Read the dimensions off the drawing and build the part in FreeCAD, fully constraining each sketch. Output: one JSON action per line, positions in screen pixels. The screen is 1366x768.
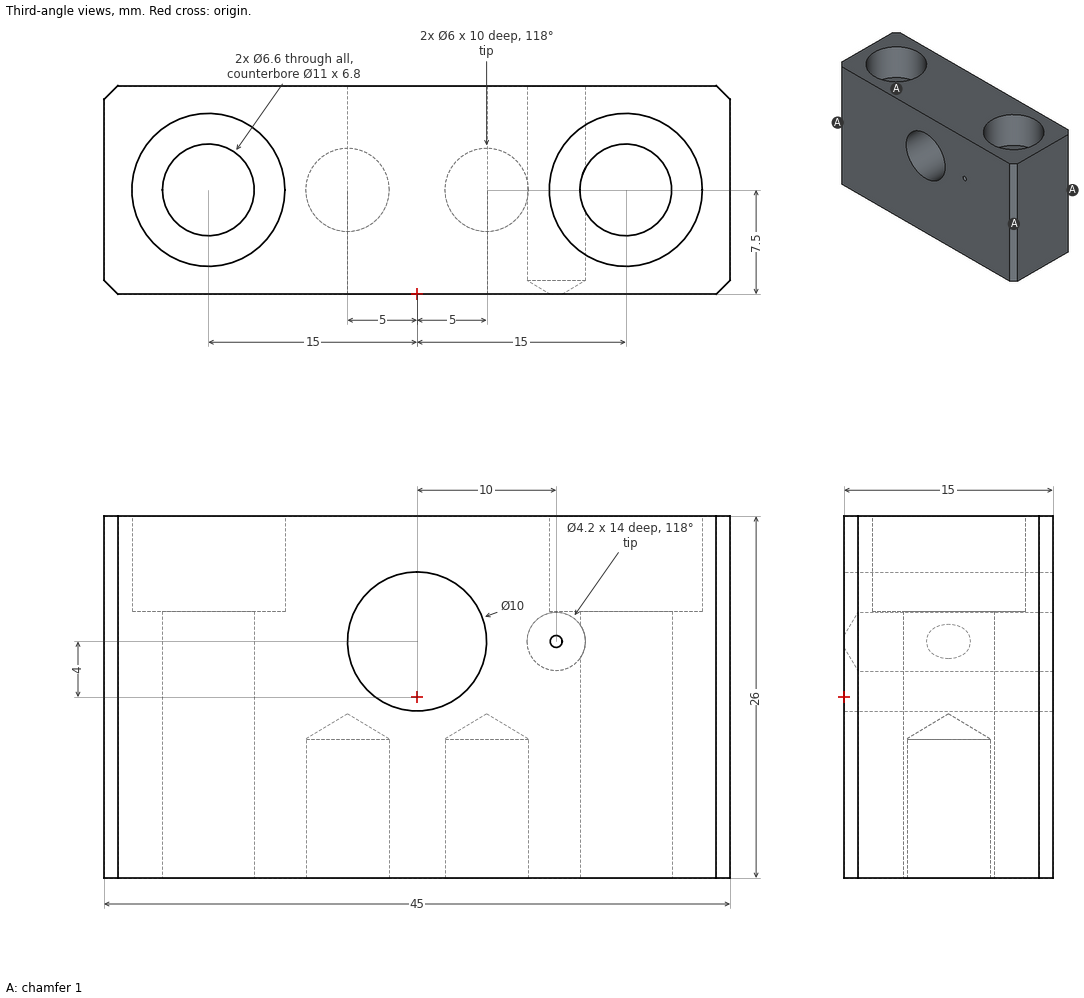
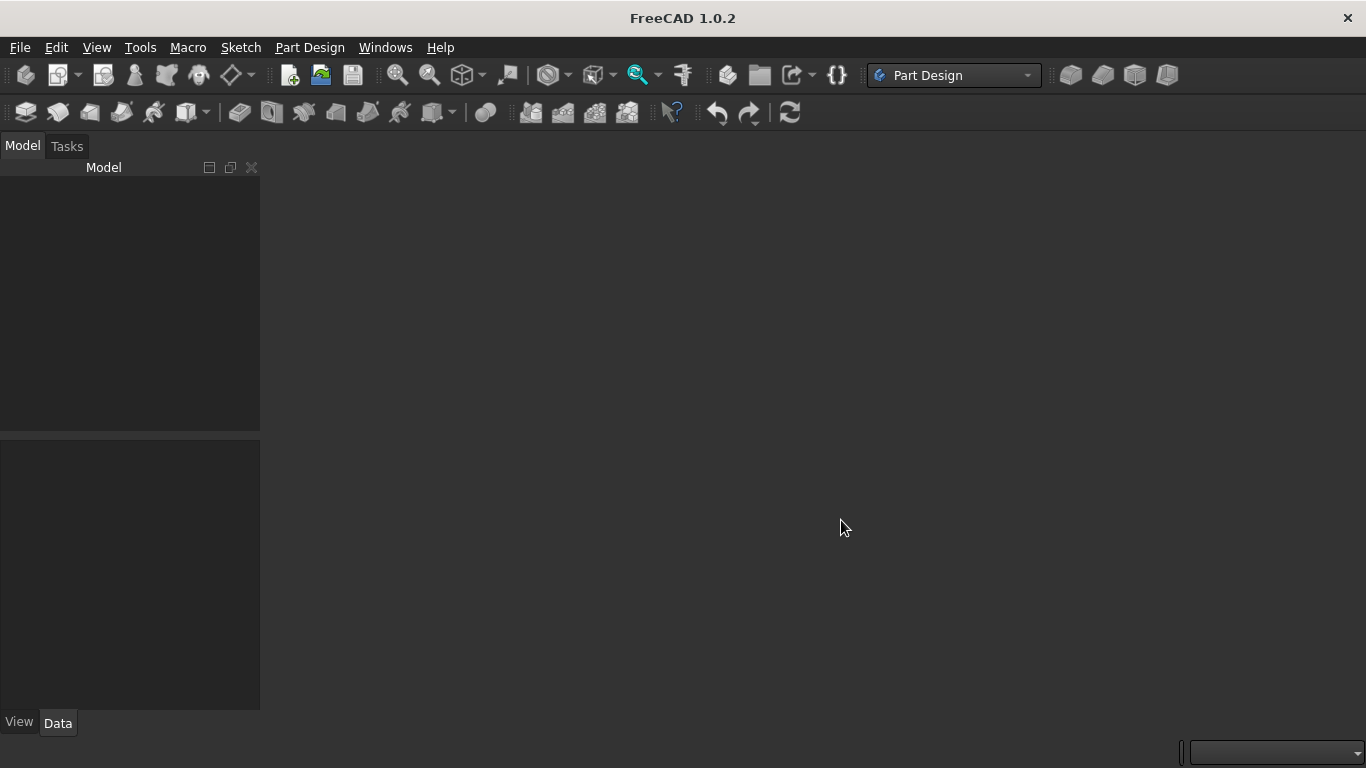
{"action": "left_click", "coordinate": [290, 76]}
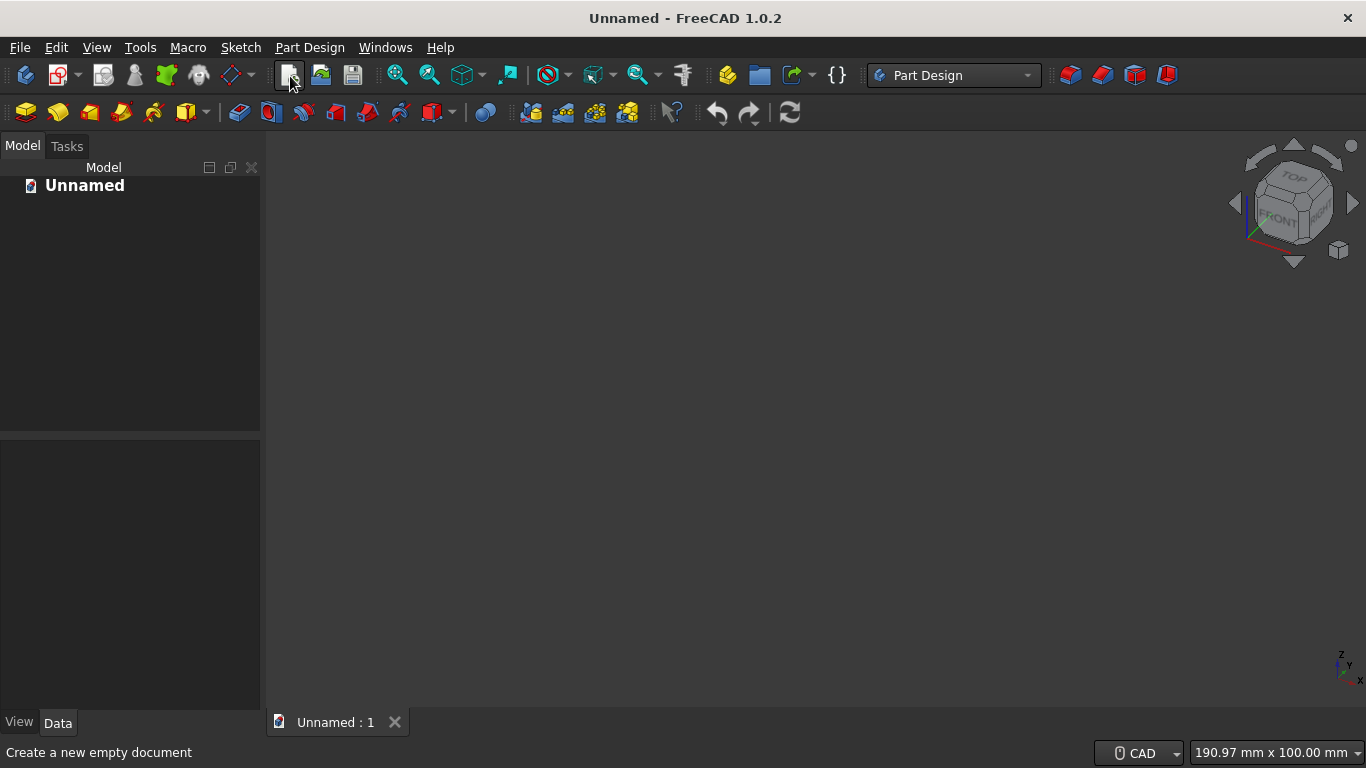
{"action": "left_click", "coordinate": [58, 76]}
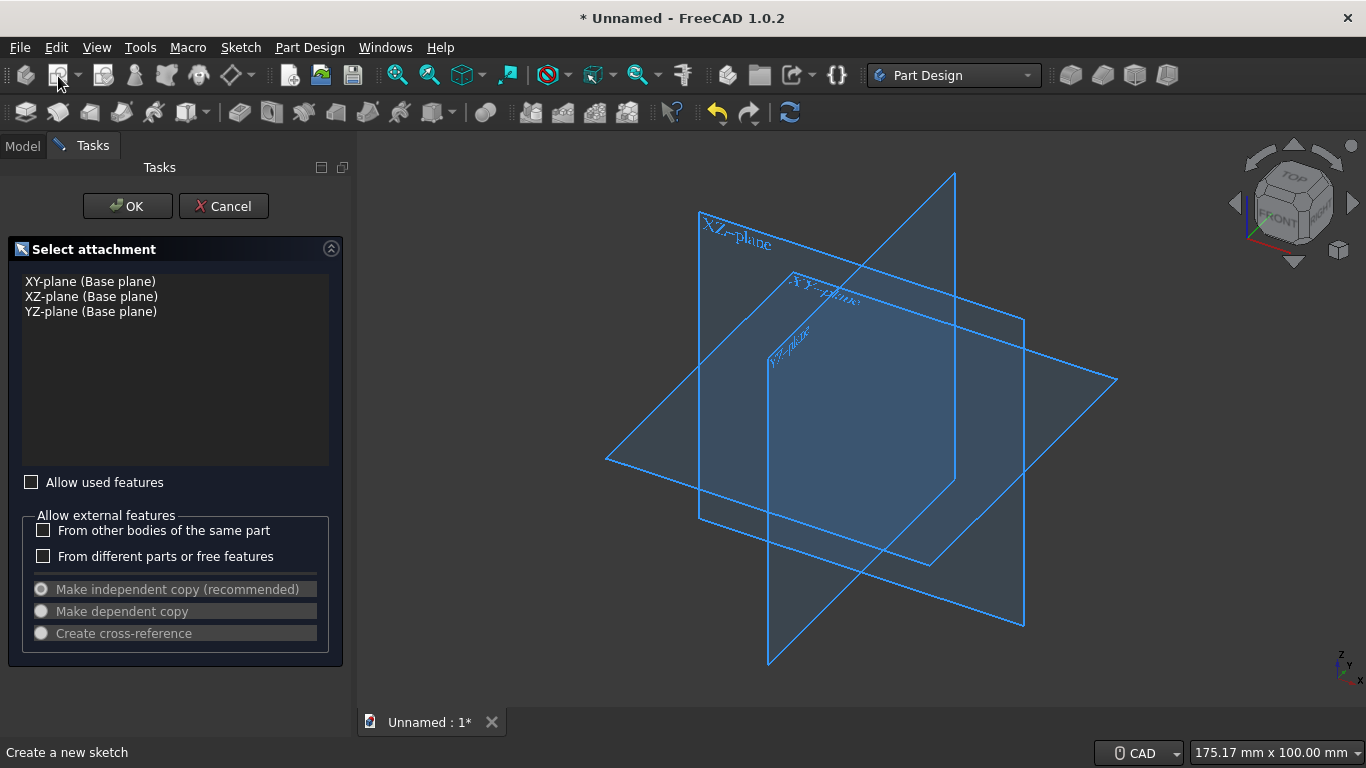
{"action": "left_click", "coordinate": [82, 296]}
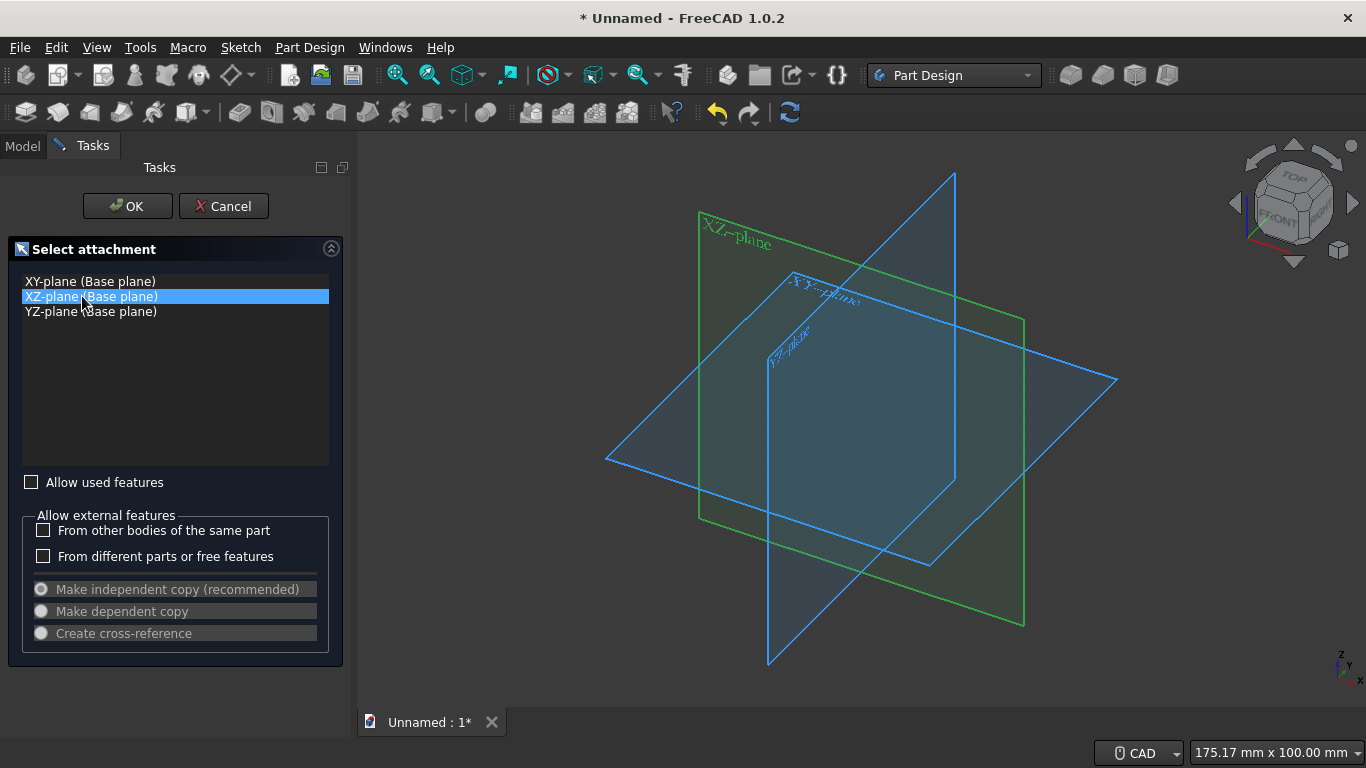
{"action": "left_click", "coordinate": [128, 206]}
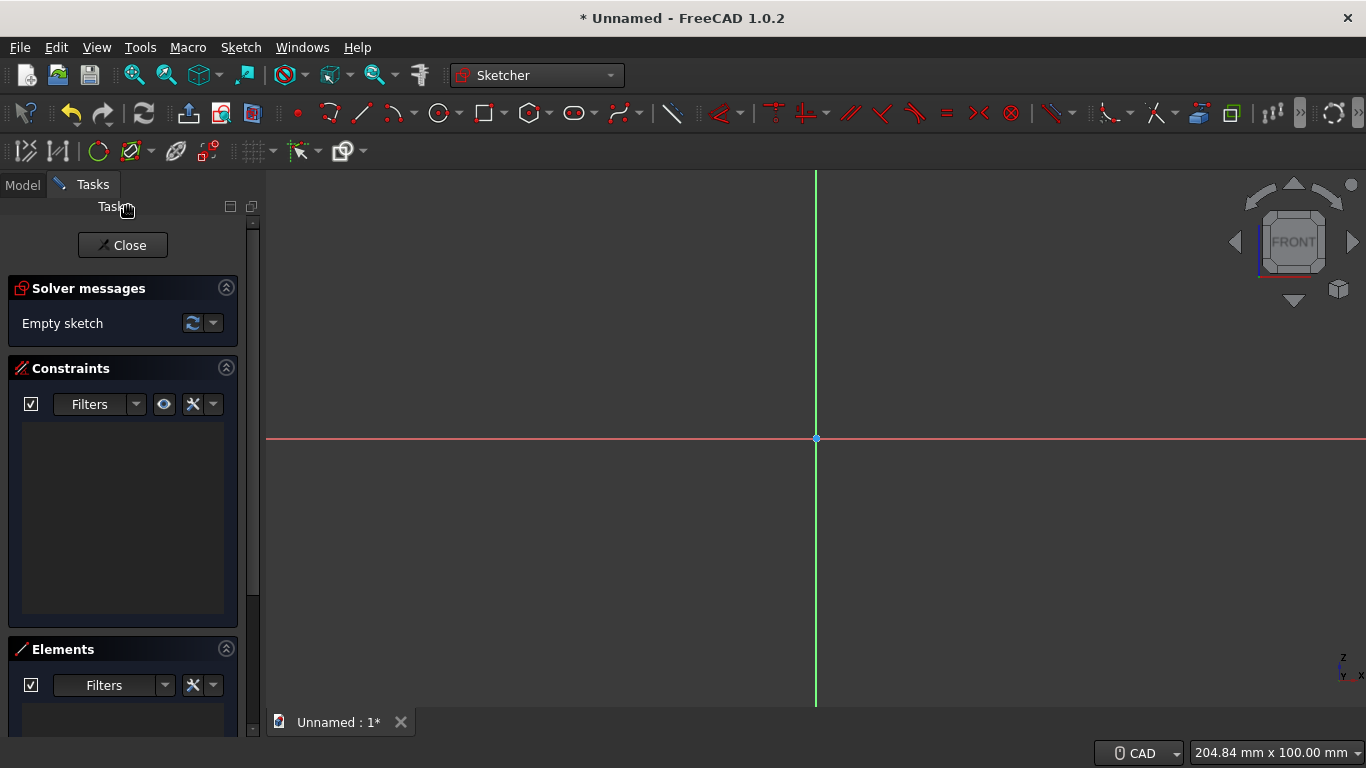
{"action": "scroll", "coordinate": [872, 438], "scroll_direction": "up", "scroll_amount": 4}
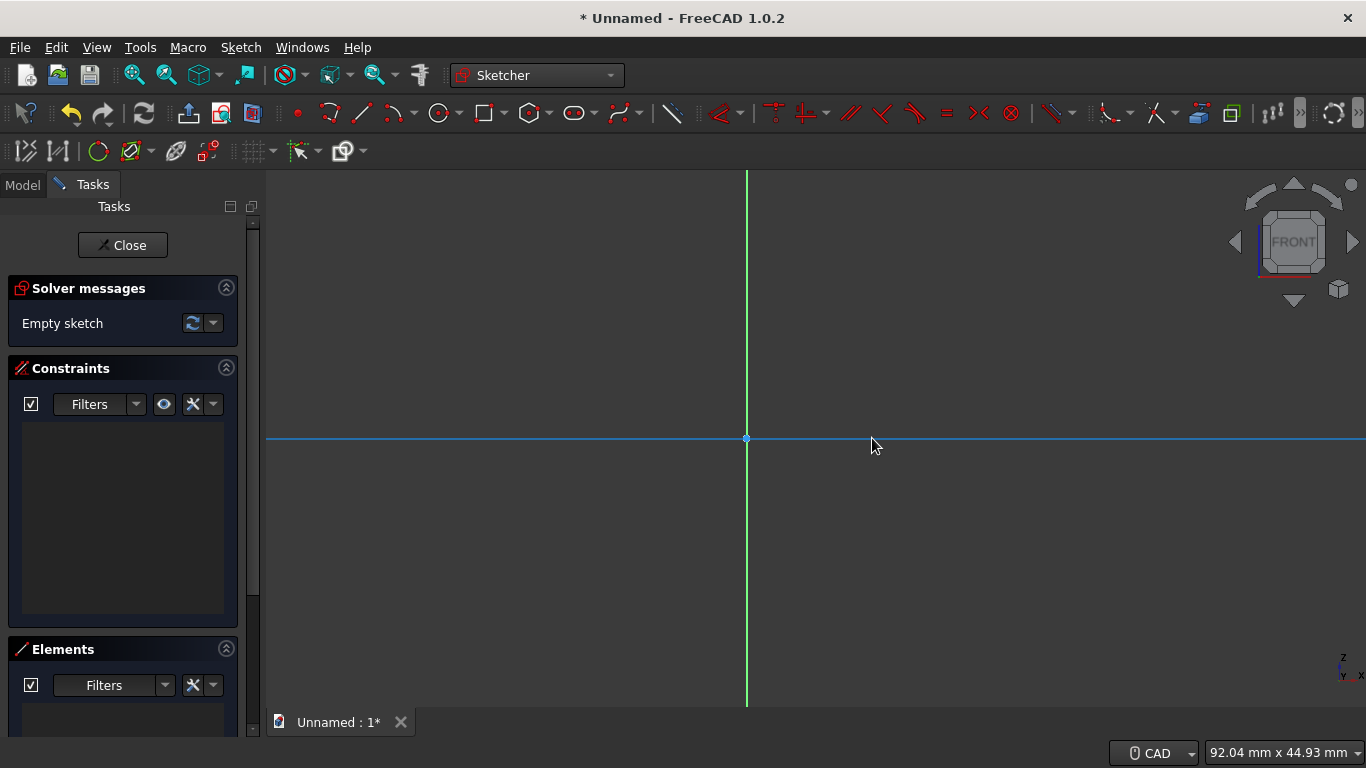
{"action": "key", "text": "g v"}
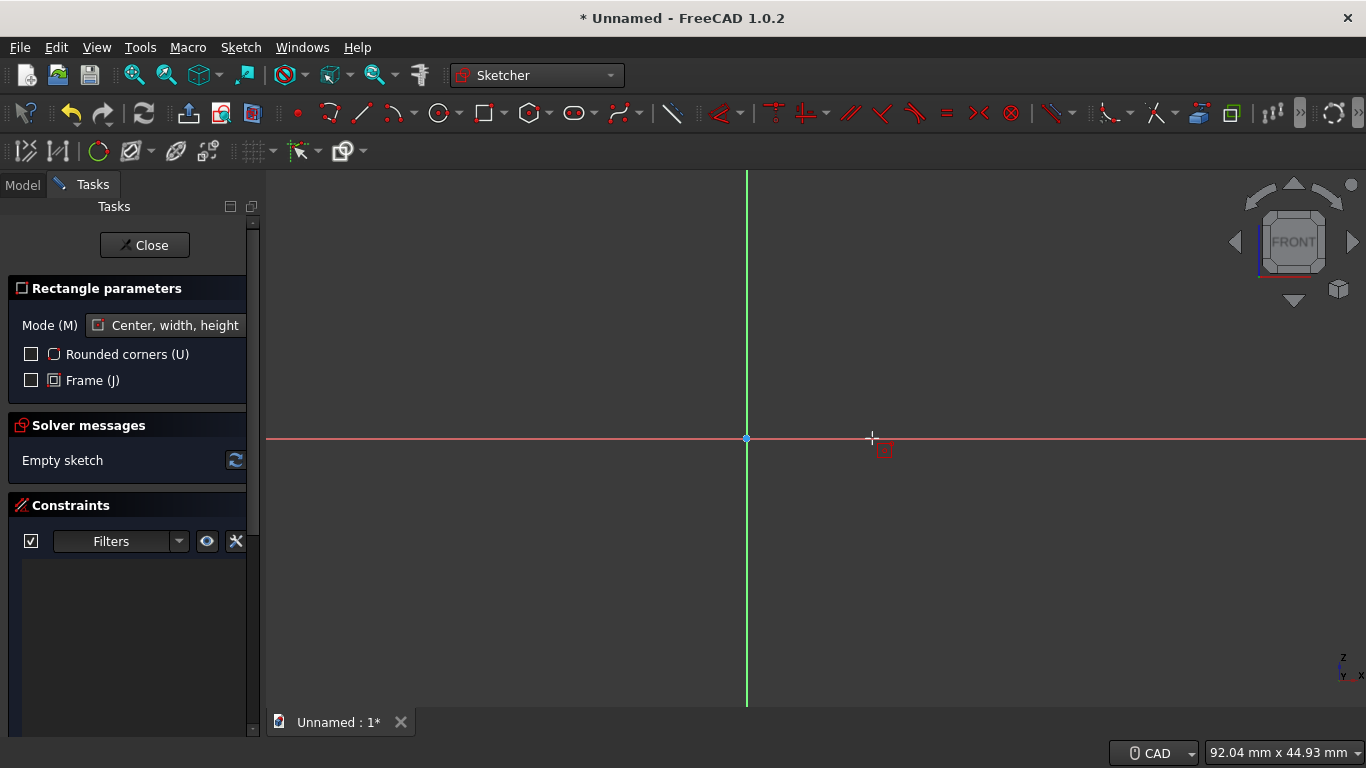
{"action": "left_click", "coordinate": [747, 438]}
{"action": "left_click", "coordinate": [1016, 283]}
{"action": "key", "text": "Escape"}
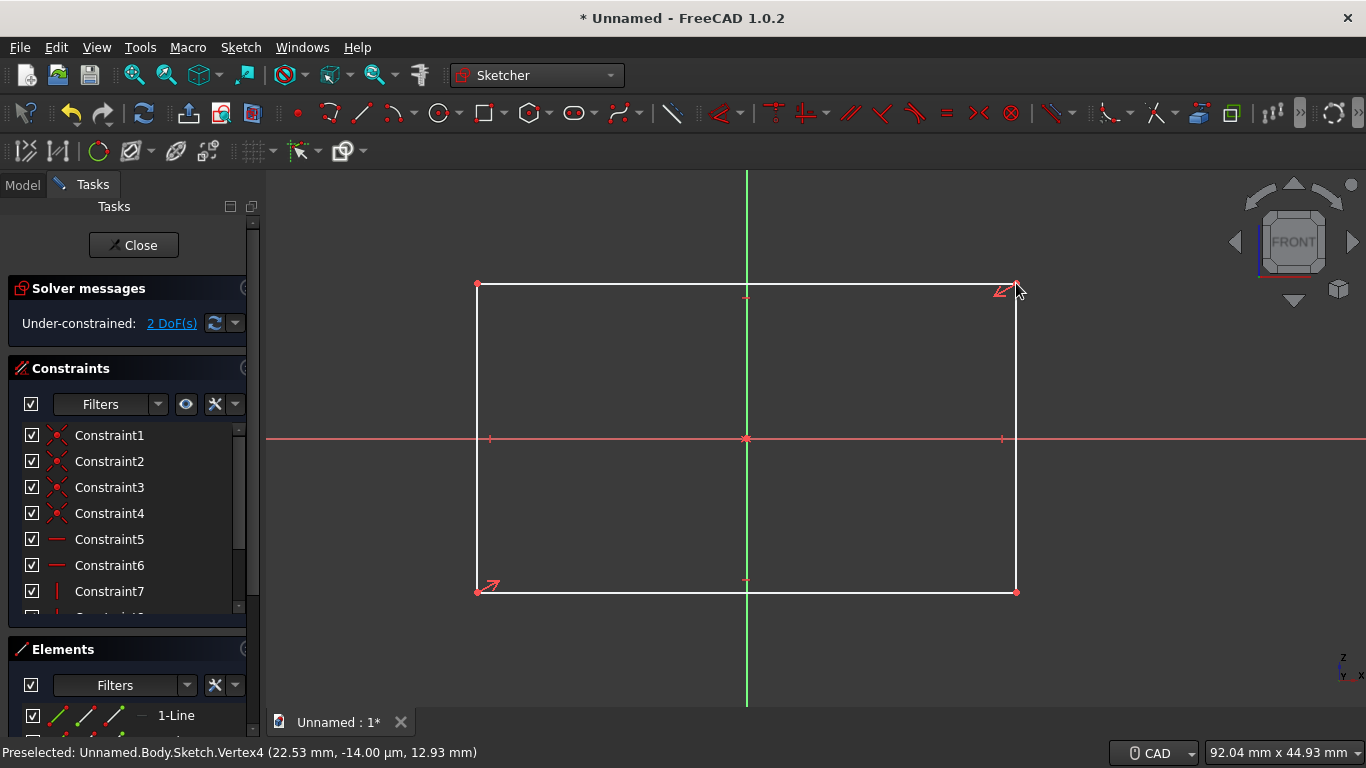
{"action": "left_click", "coordinate": [720, 114]}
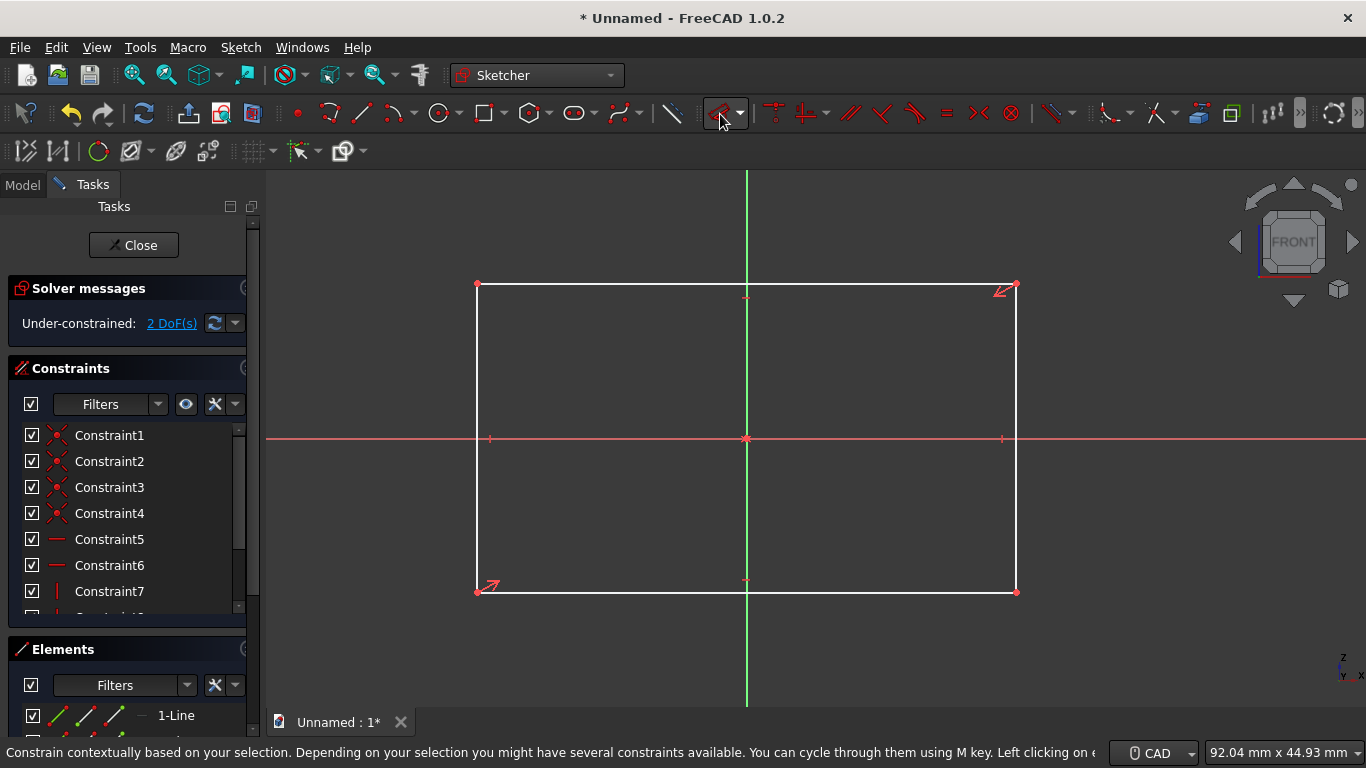
{"action": "left_click", "coordinate": [639, 593]}
{"action": "left_click", "coordinate": [623, 627]}